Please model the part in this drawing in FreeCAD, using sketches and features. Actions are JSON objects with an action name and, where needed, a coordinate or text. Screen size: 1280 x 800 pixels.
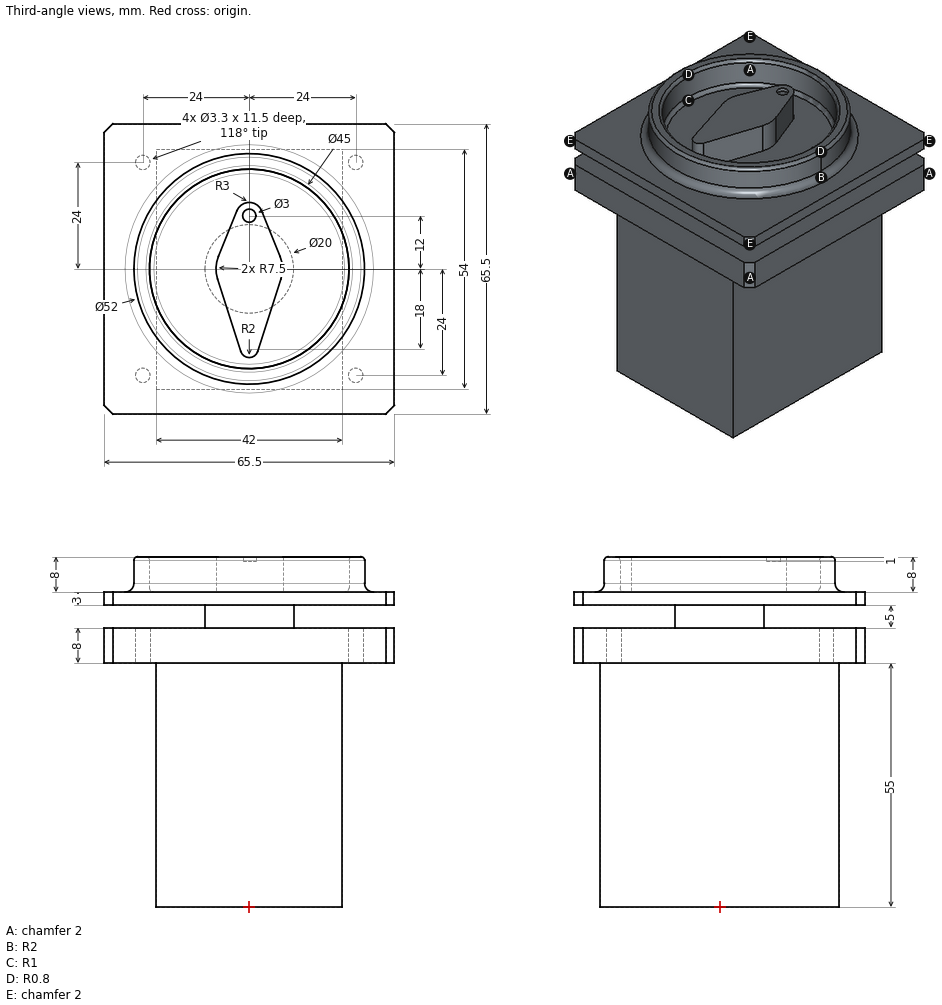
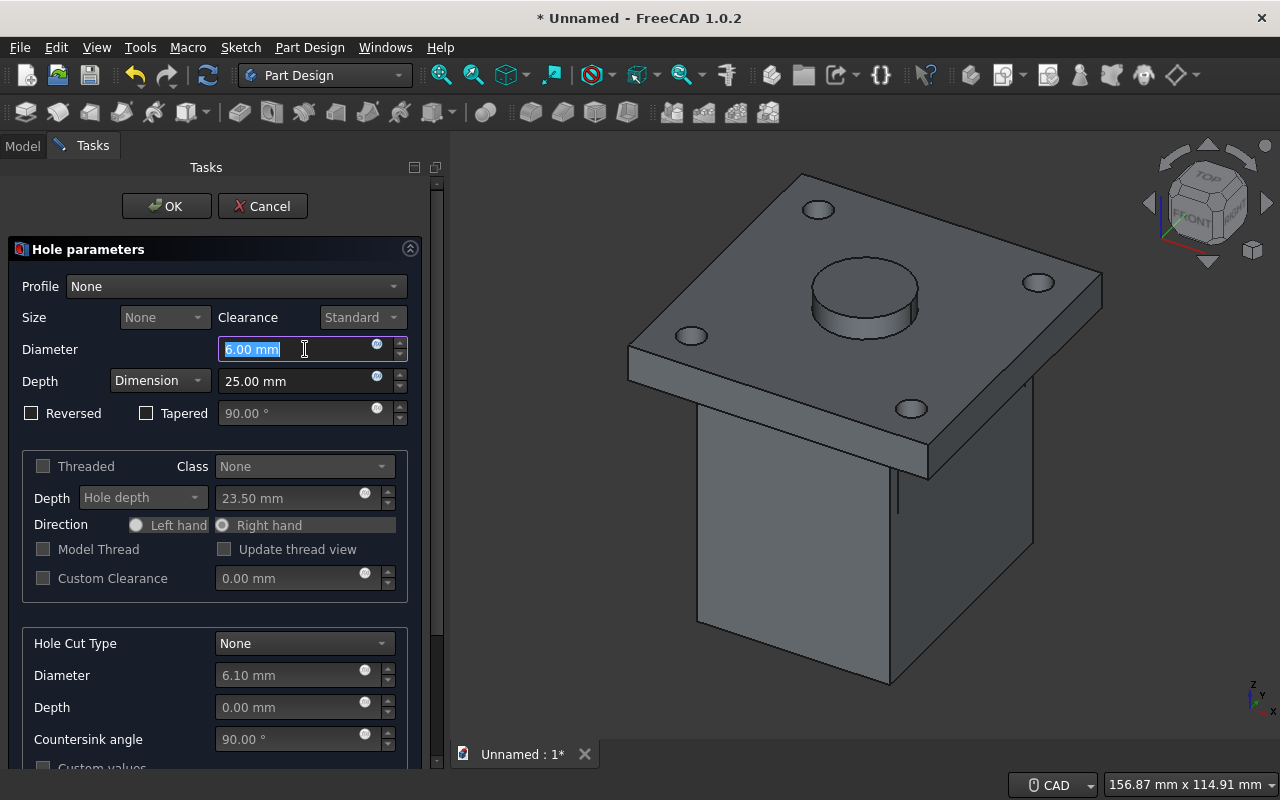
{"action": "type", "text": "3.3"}
{"action": "key", "text": "Tab"}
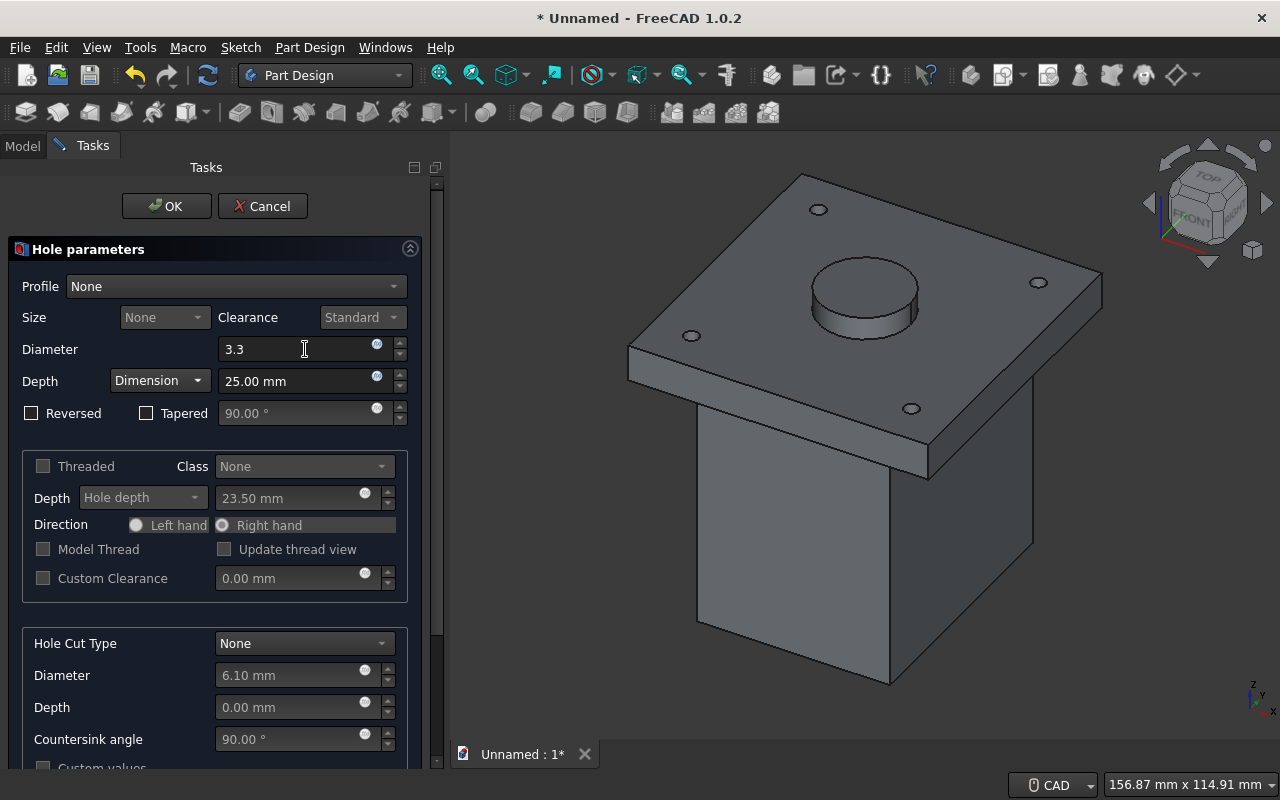
{"action": "triple_click", "coordinate": [305, 381]}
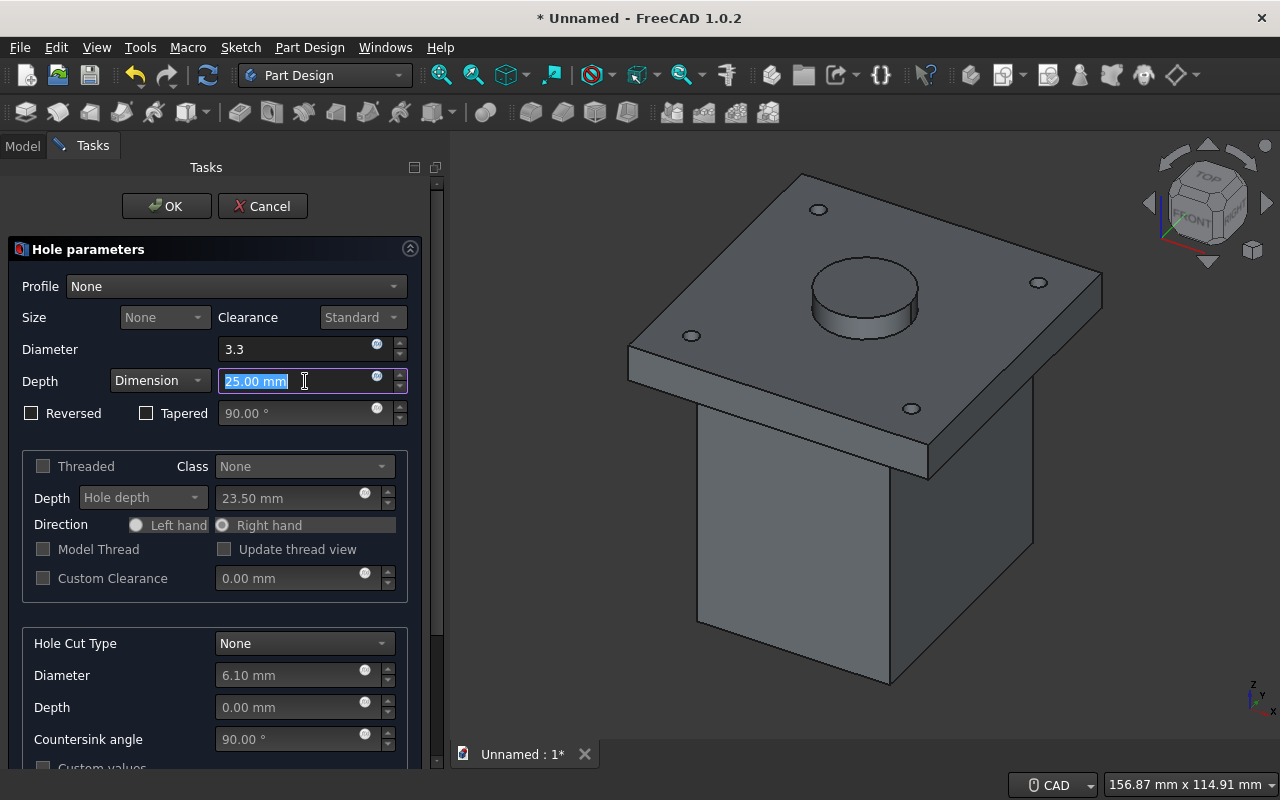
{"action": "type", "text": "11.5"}
{"action": "key", "text": "Tab"}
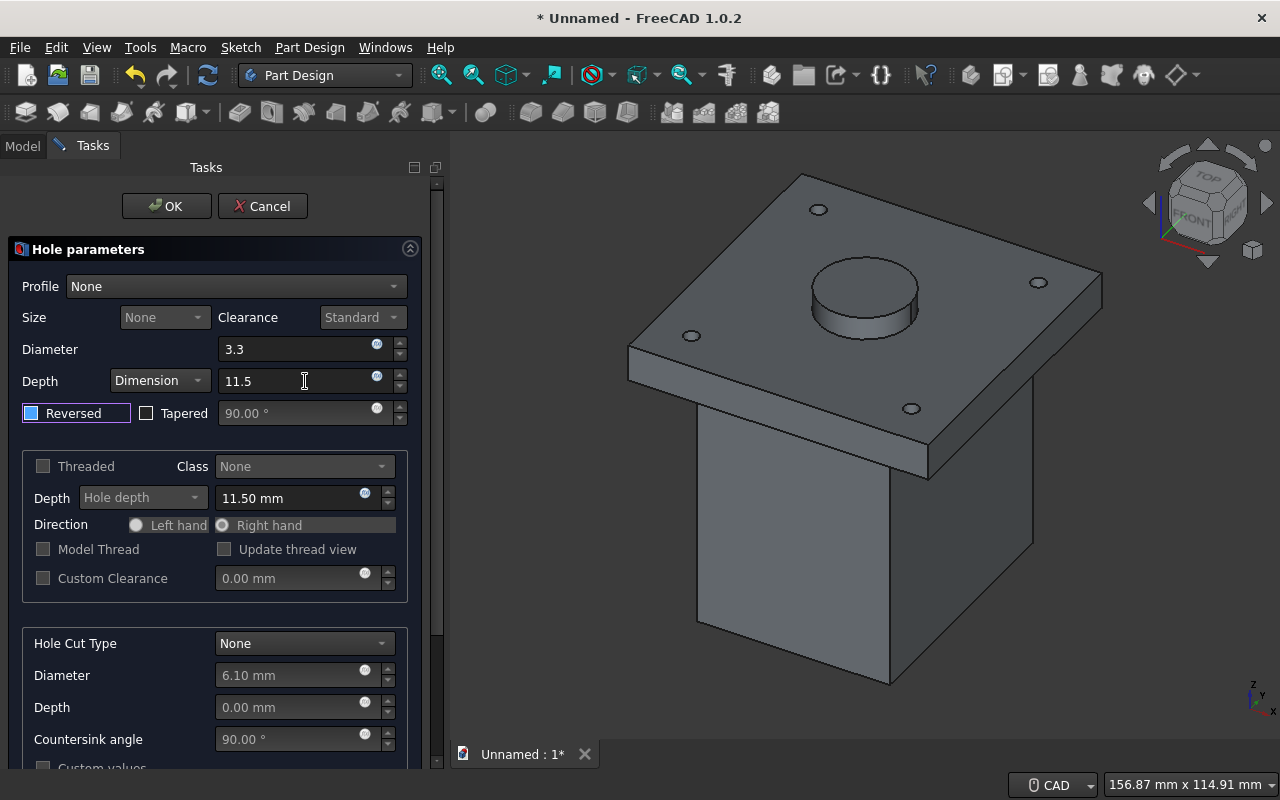
{"action": "left_click", "coordinate": [167, 206]}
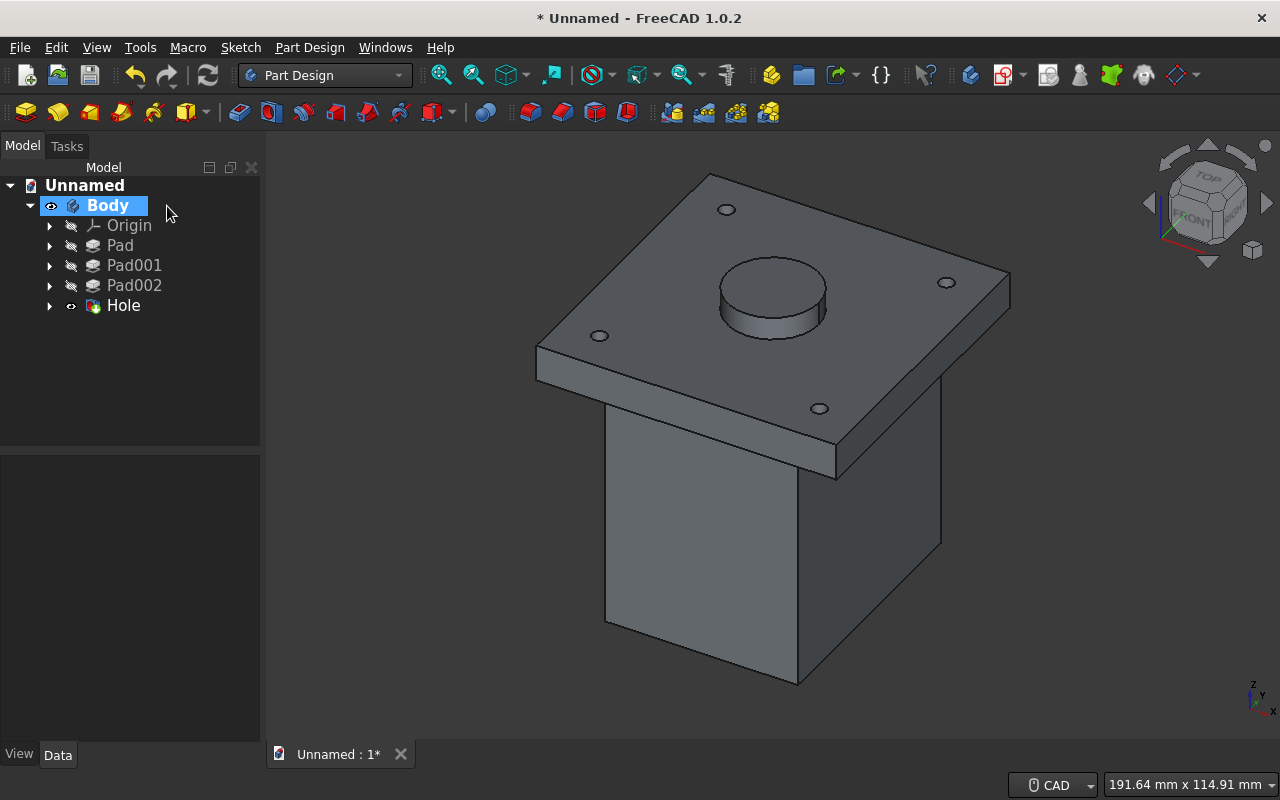
{"action": "left_click", "coordinate": [836, 461]}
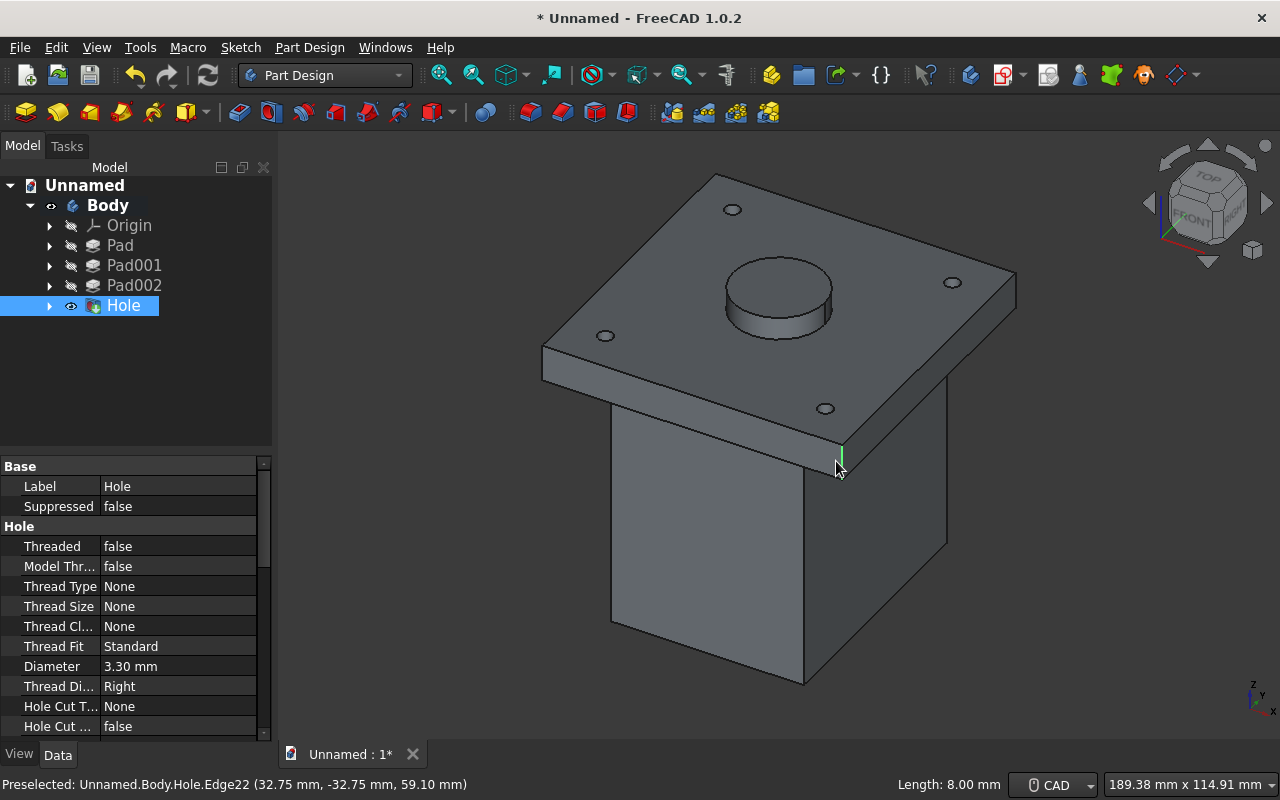
{"action": "key", "text": "0"}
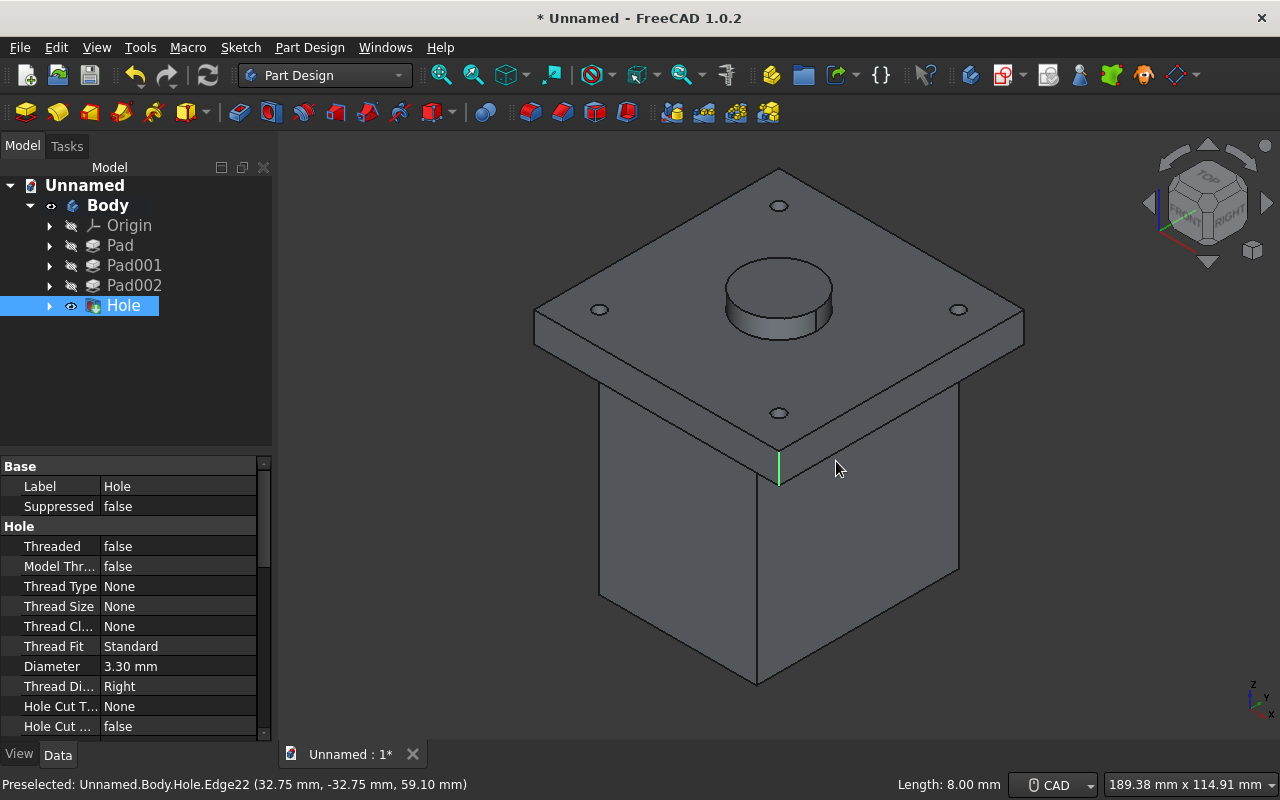
{"action": "key", "text": "2"}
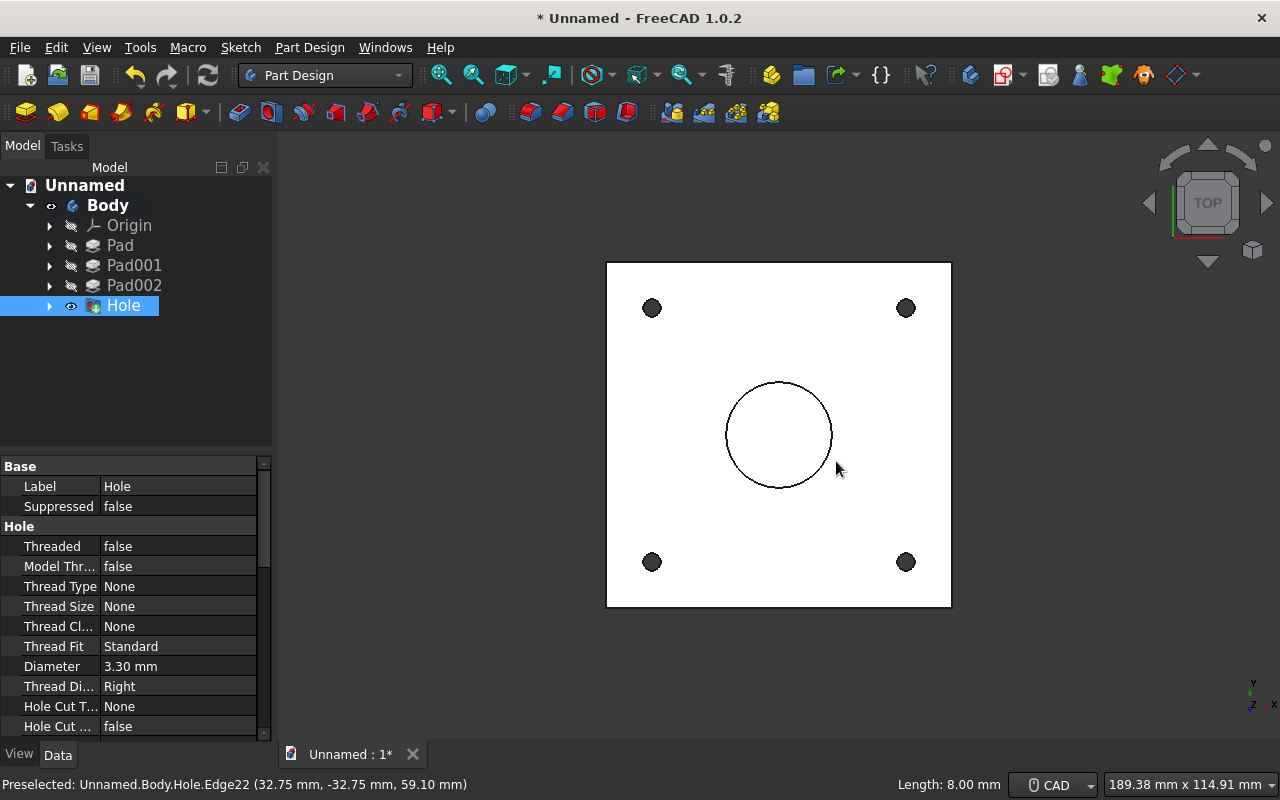
{"action": "key", "text": "1"}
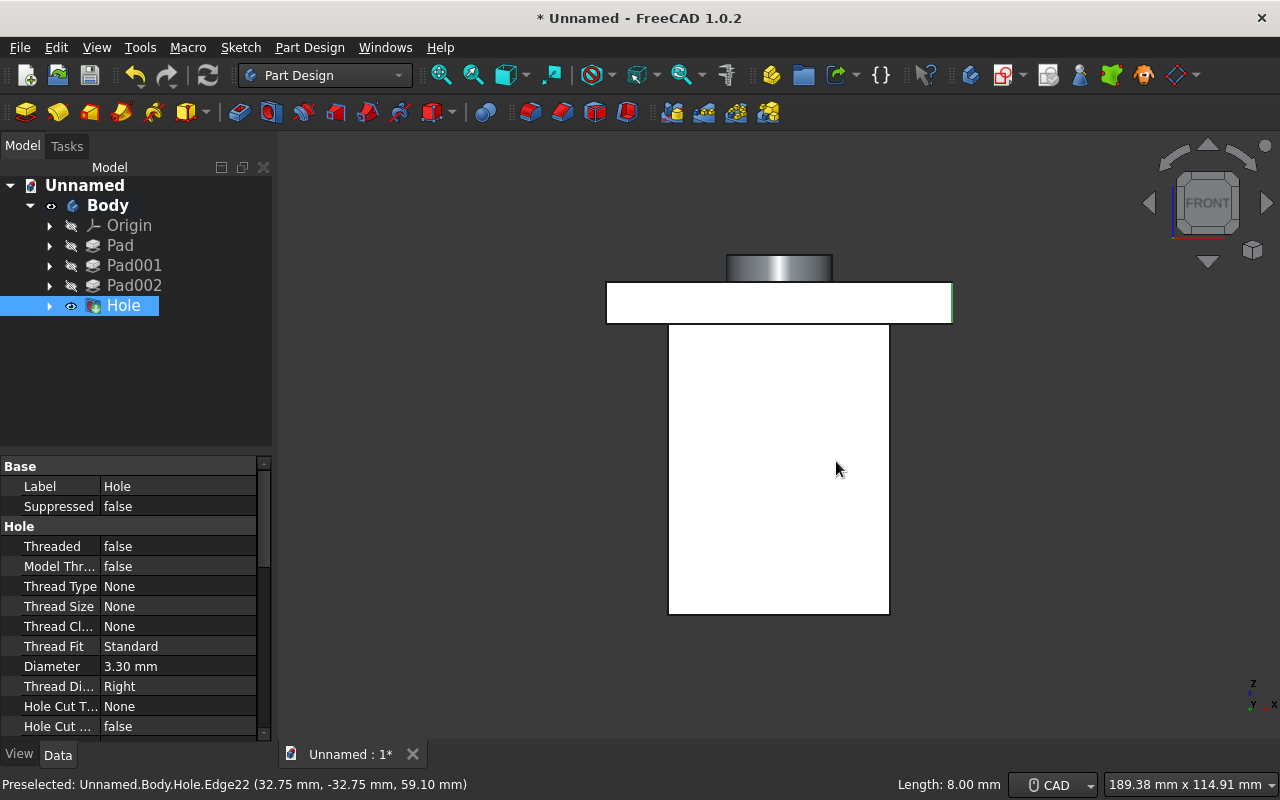
{"action": "left_click", "coordinate": [606, 302], "text": "ctrl"}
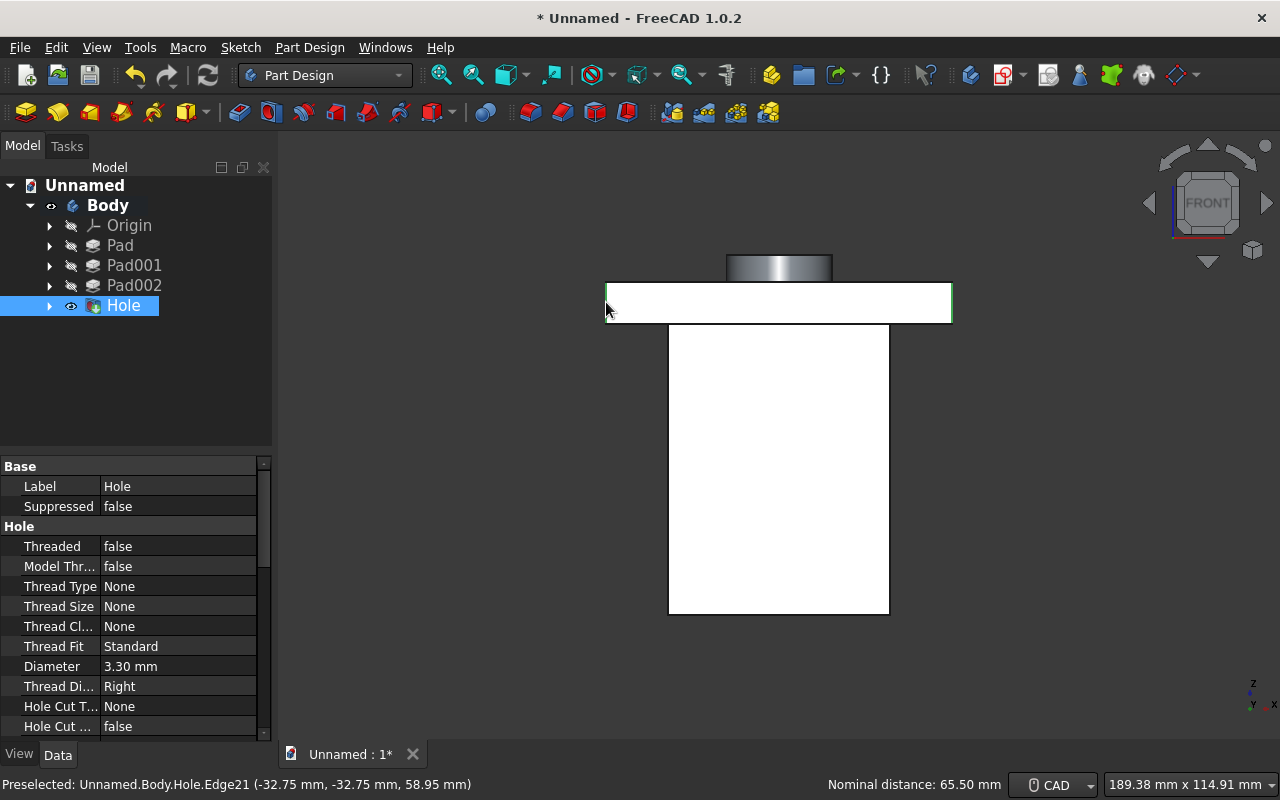
{"action": "key", "text": "3"}